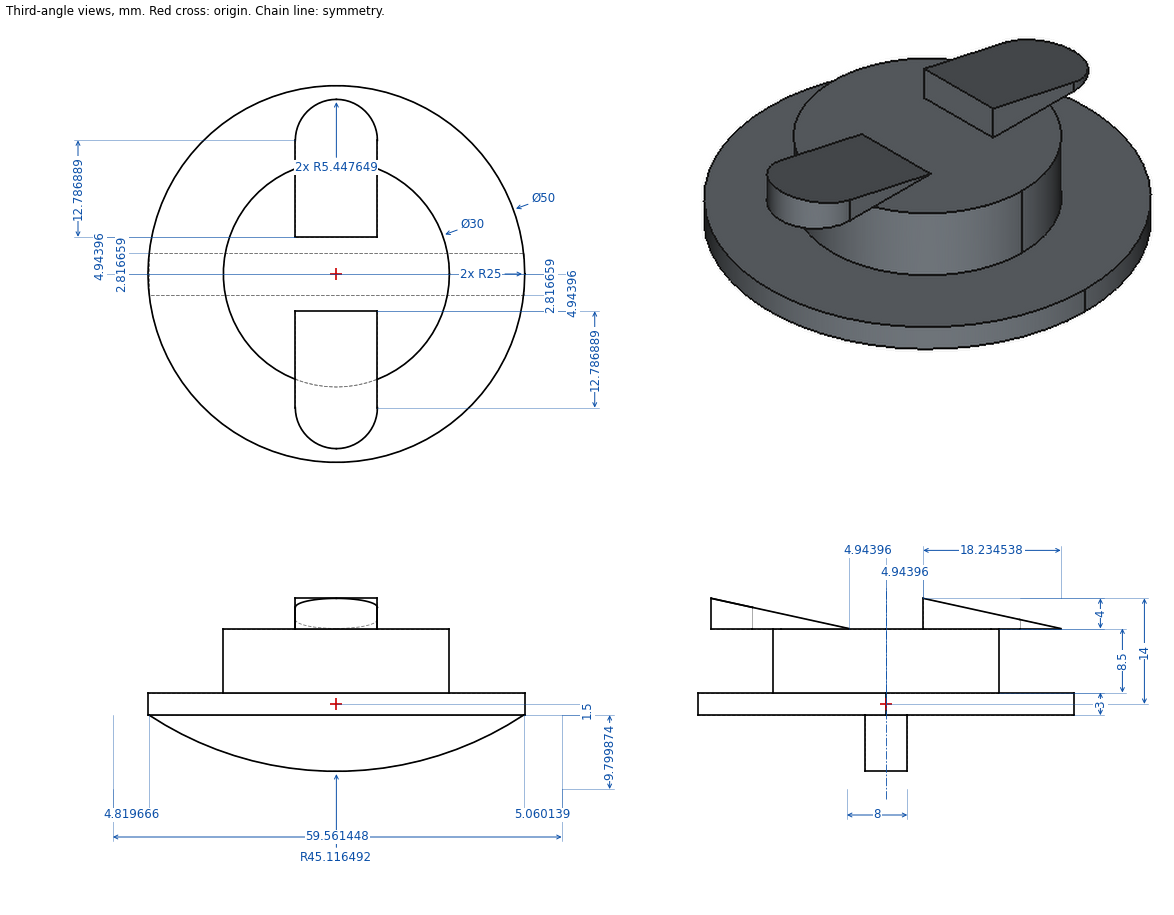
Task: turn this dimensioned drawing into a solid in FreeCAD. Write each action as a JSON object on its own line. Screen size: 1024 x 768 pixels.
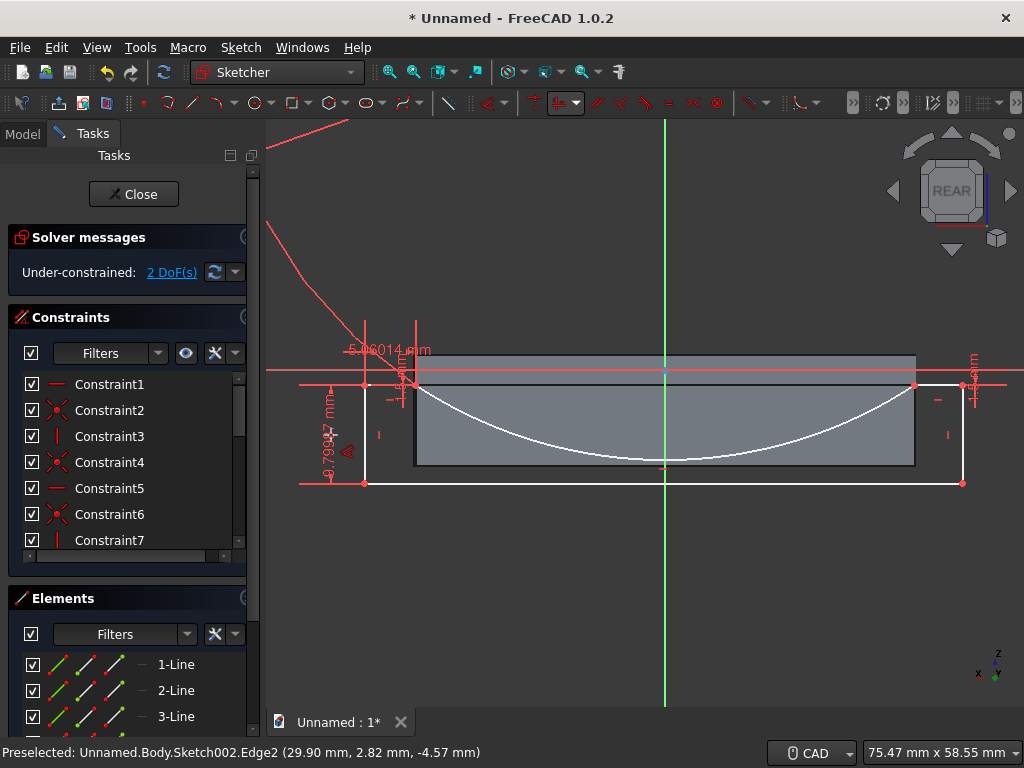
{"action": "scroll", "coordinate": [399, 385], "scroll_direction": "down", "scroll_amount": 2}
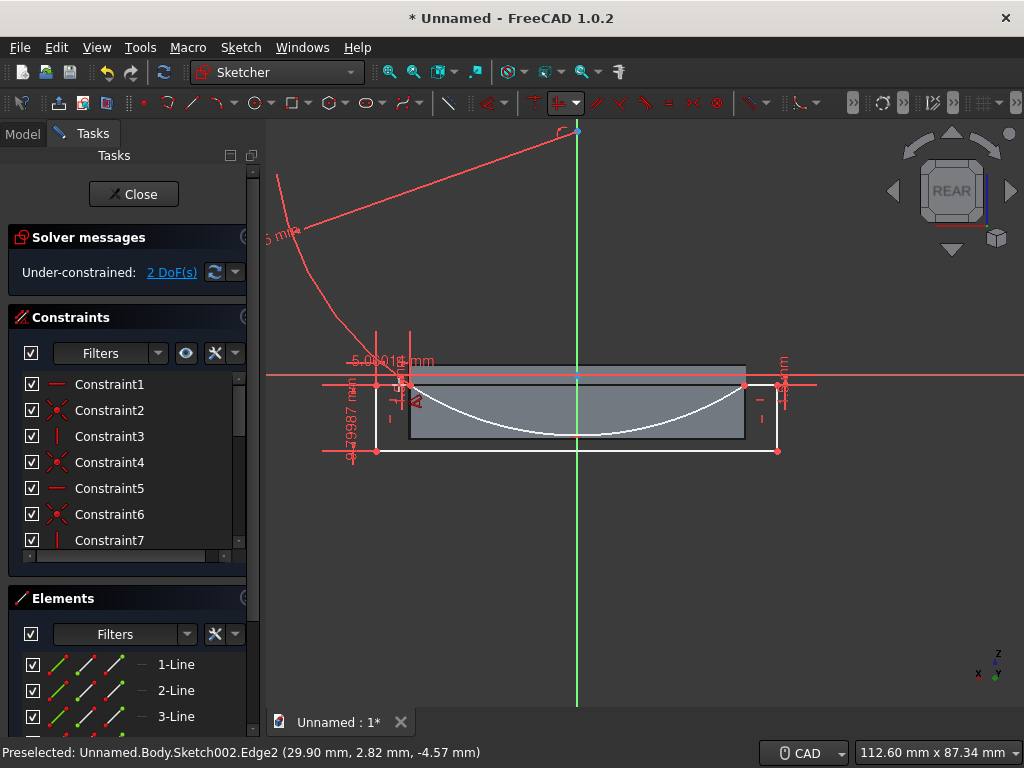
{"action": "scroll", "coordinate": [767, 385], "scroll_direction": "up", "scroll_amount": 2}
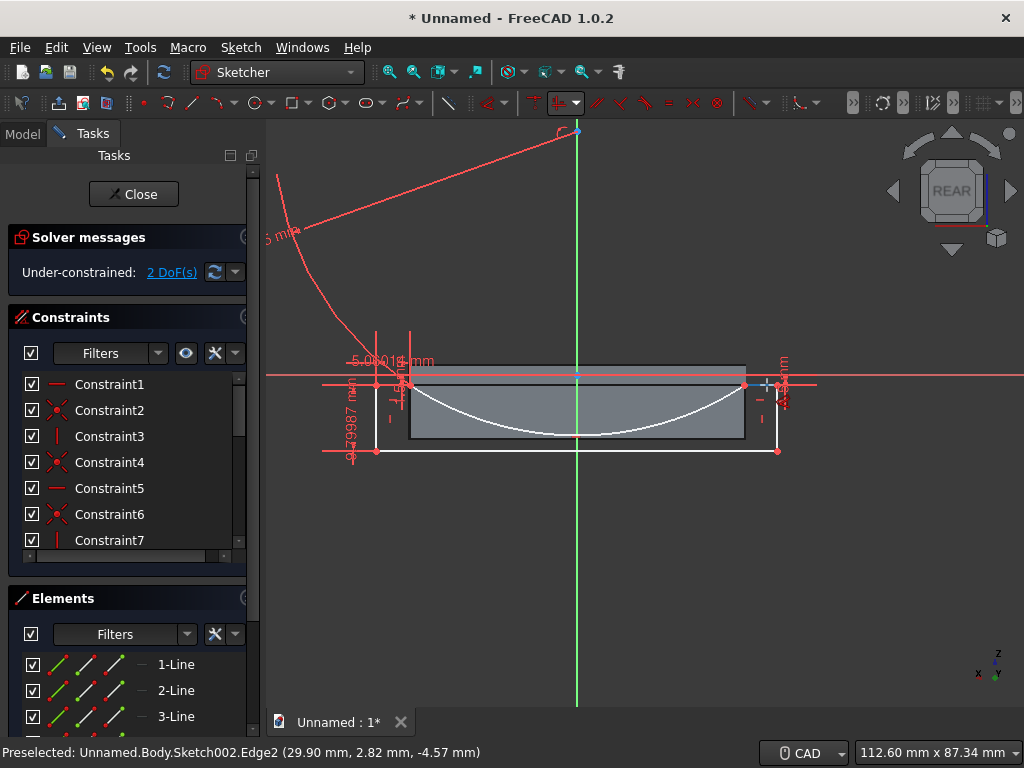
{"action": "left_click", "coordinate": [767, 385]}
{"action": "left_click", "coordinate": [758, 351]}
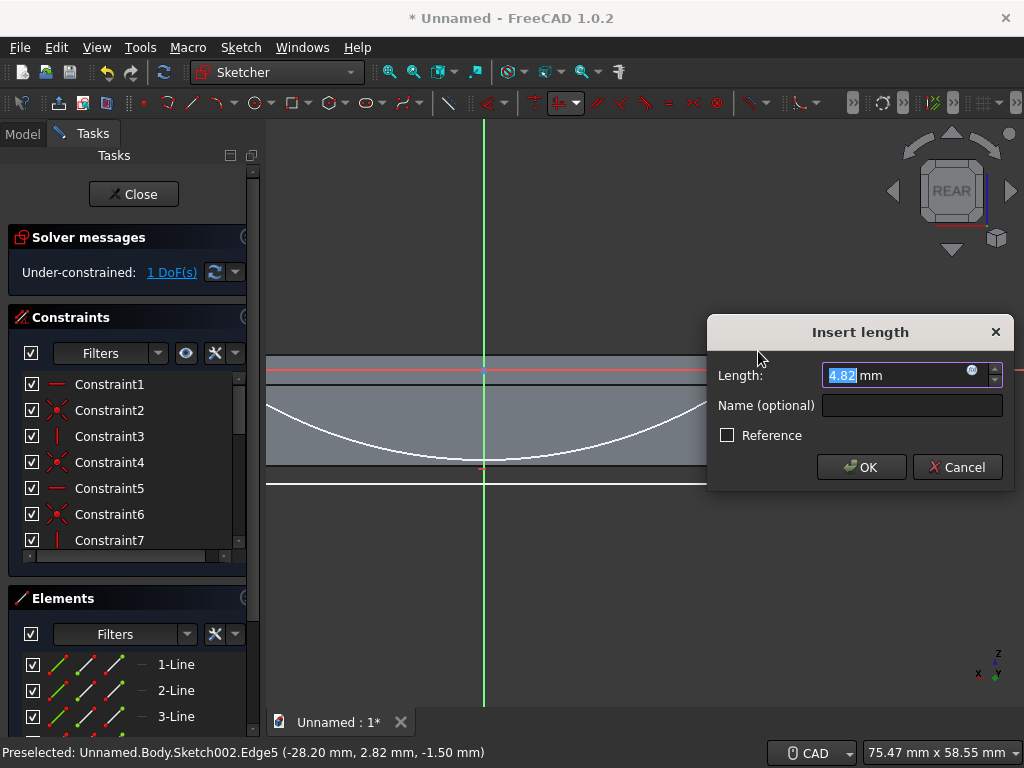
{"action": "type", "text": "4.819666"}
{"action": "key", "text": "Return"}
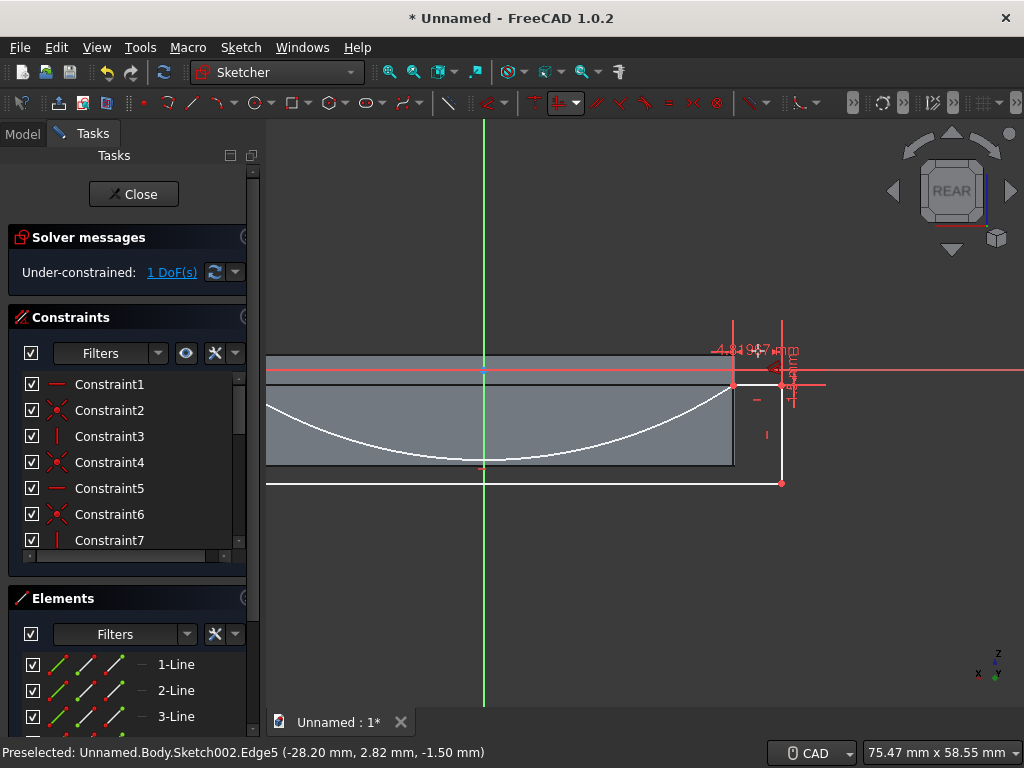
{"action": "left_click", "coordinate": [363, 484]}
{"action": "left_click", "coordinate": [538, 518]}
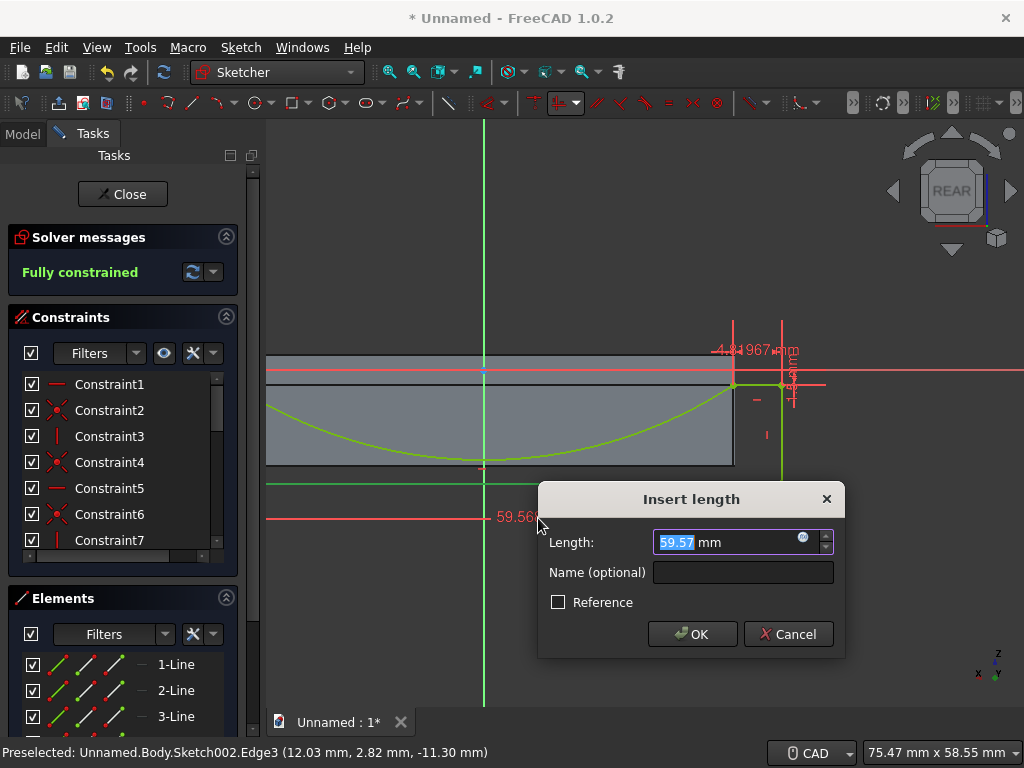
{"action": "type", "text": "59.561448"}
{"action": "key", "text": "Return"}
{"action": "key", "text": "Escape"}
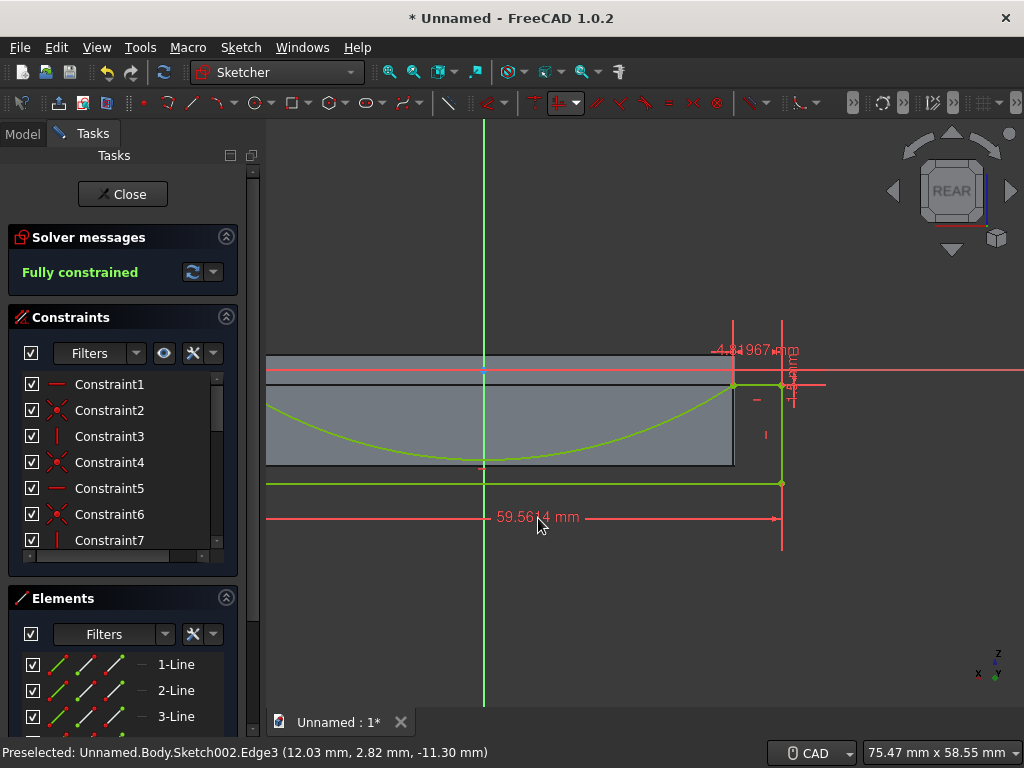
{"action": "left_click", "coordinate": [123, 194]}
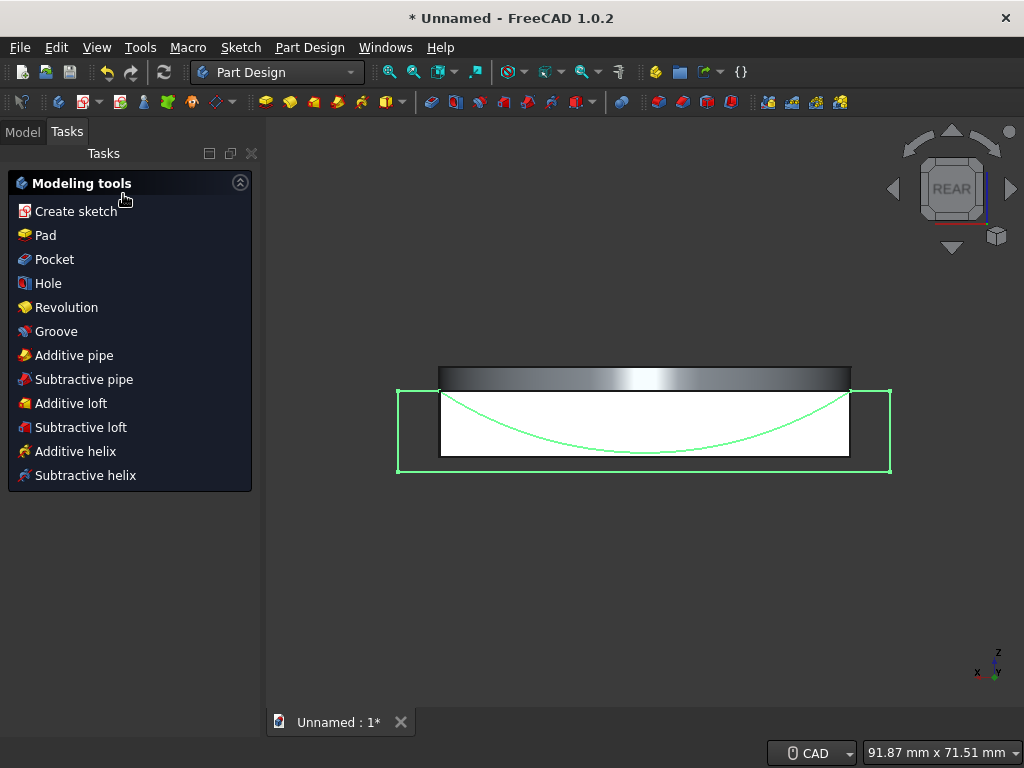
{"action": "left_click", "coordinate": [432, 102]}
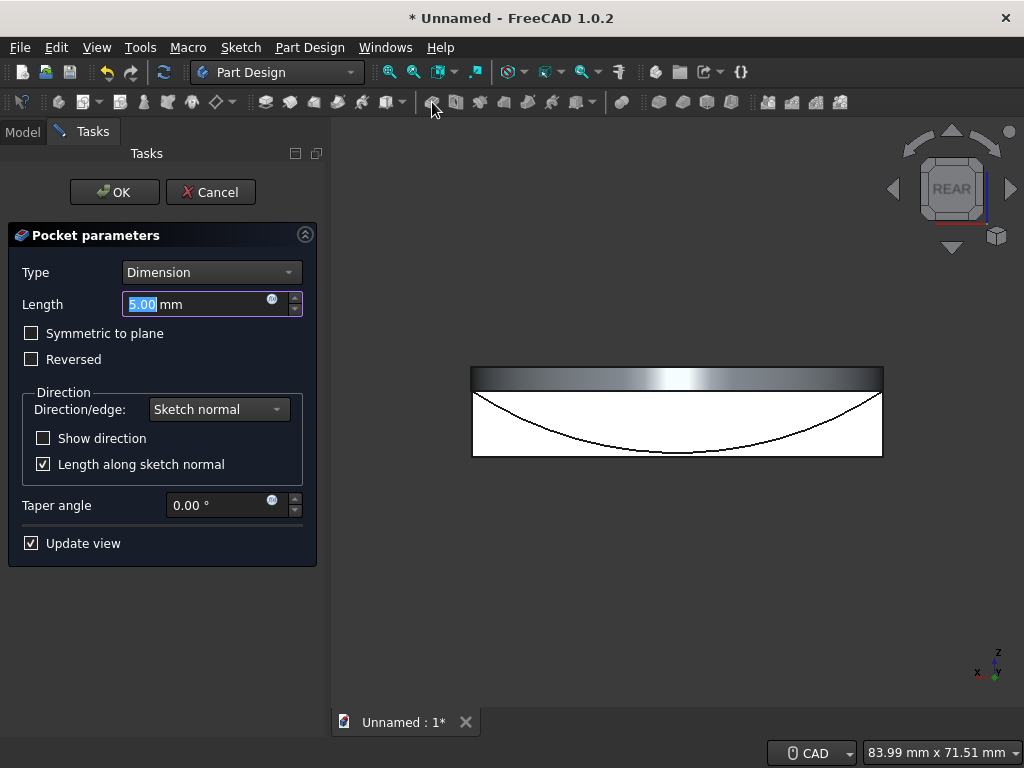
{"action": "type", "text": "8"}
{"action": "key", "text": "Tab"}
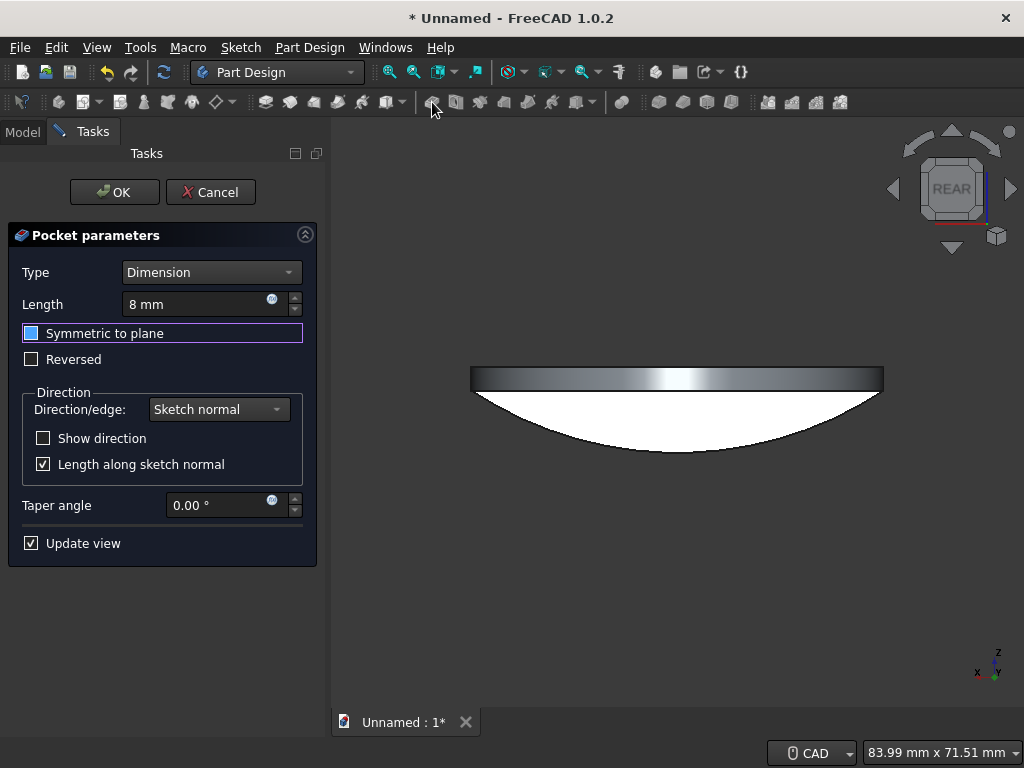
{"action": "left_click", "coordinate": [115, 192]}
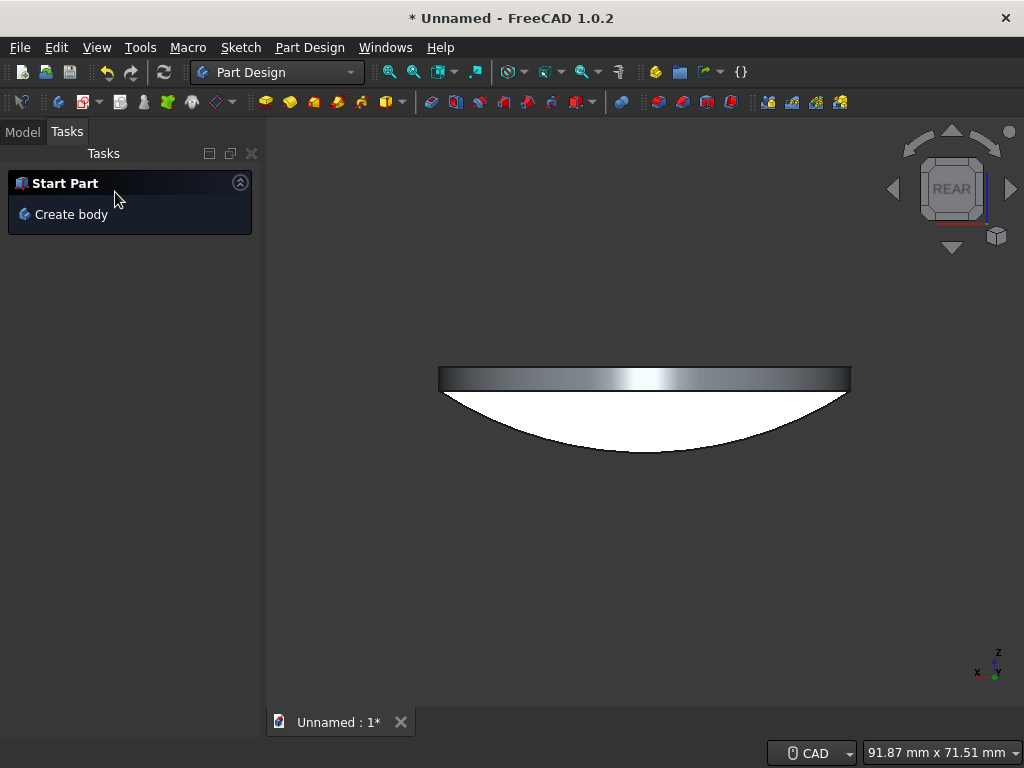
{"action": "key", "text": "0"}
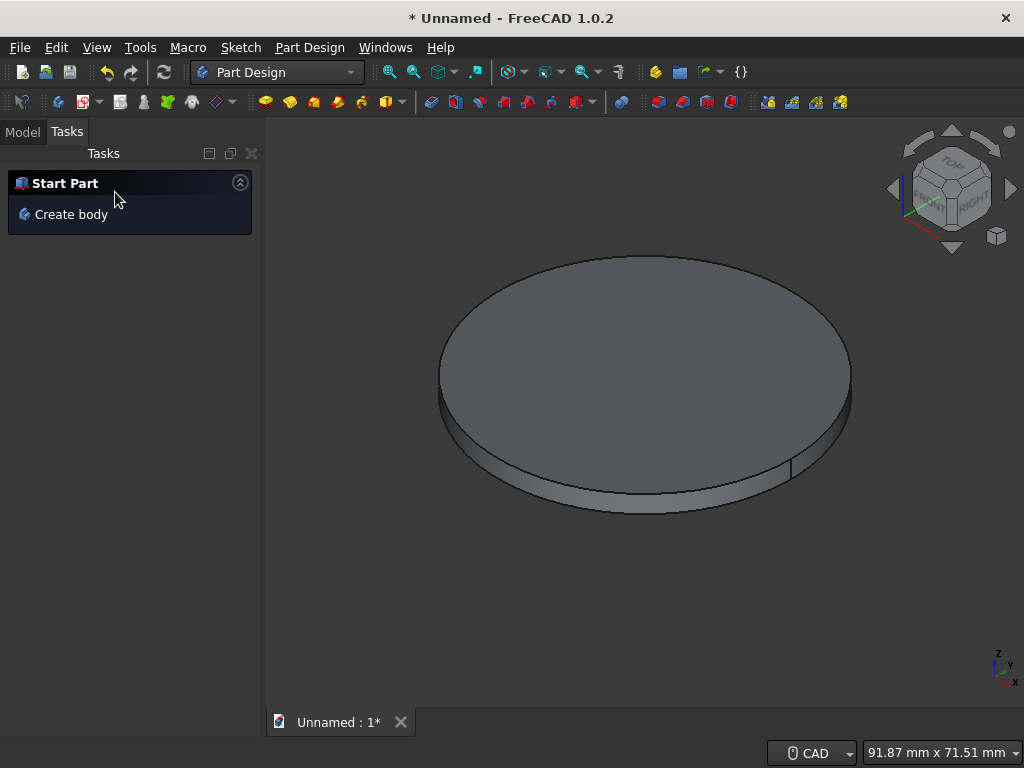
{"action": "left_click", "coordinate": [645, 374]}